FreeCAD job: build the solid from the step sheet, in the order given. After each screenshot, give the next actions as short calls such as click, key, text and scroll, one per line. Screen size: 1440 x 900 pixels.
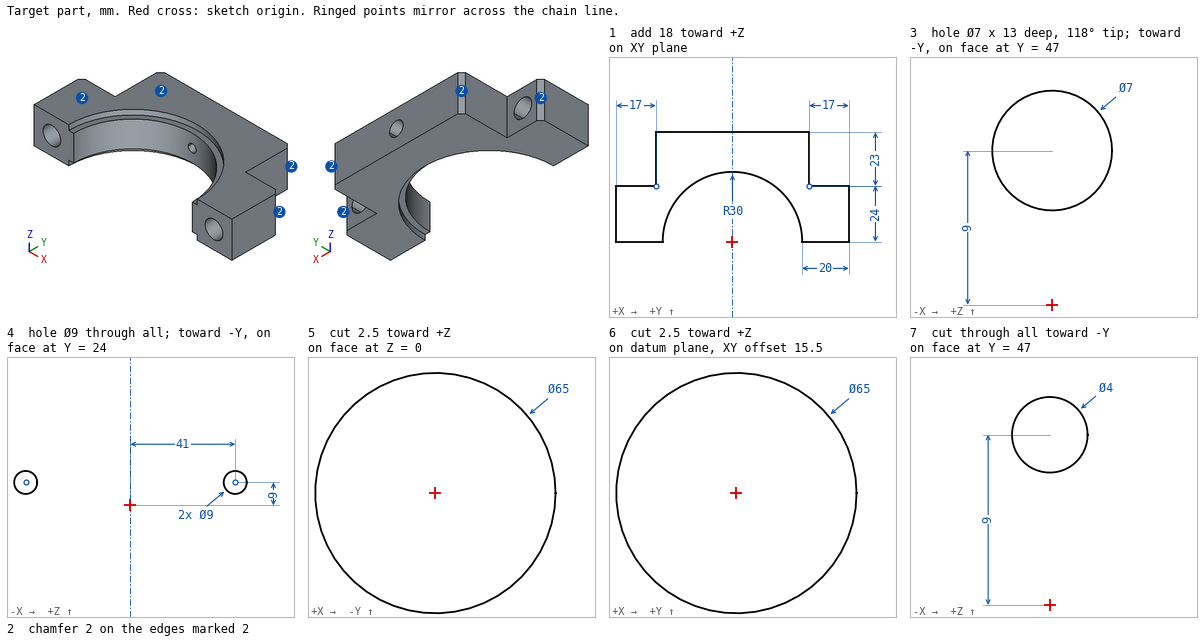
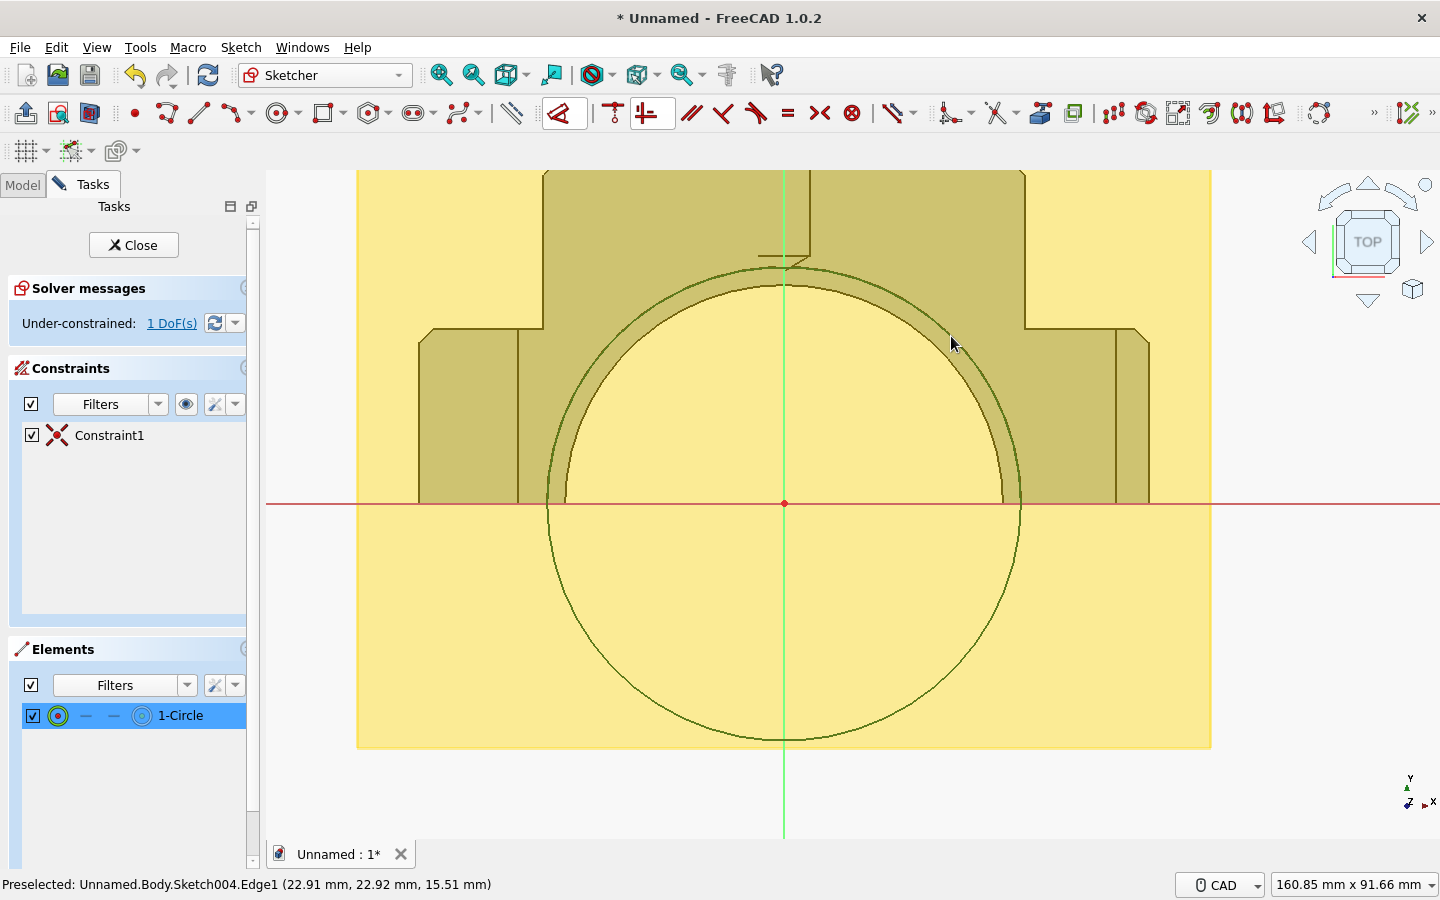
click(582, 114)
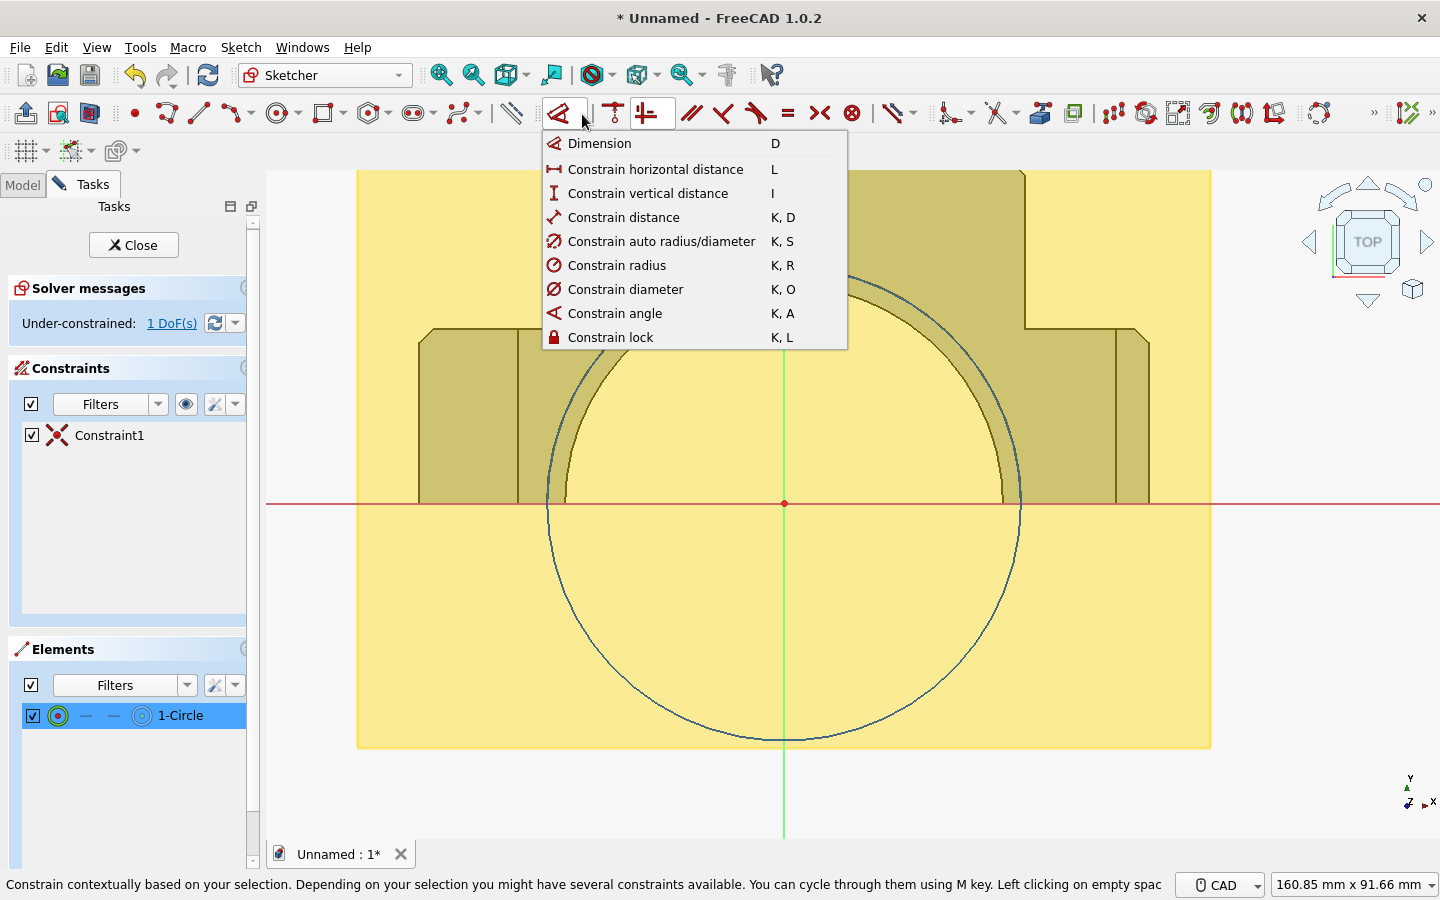
click(695, 289)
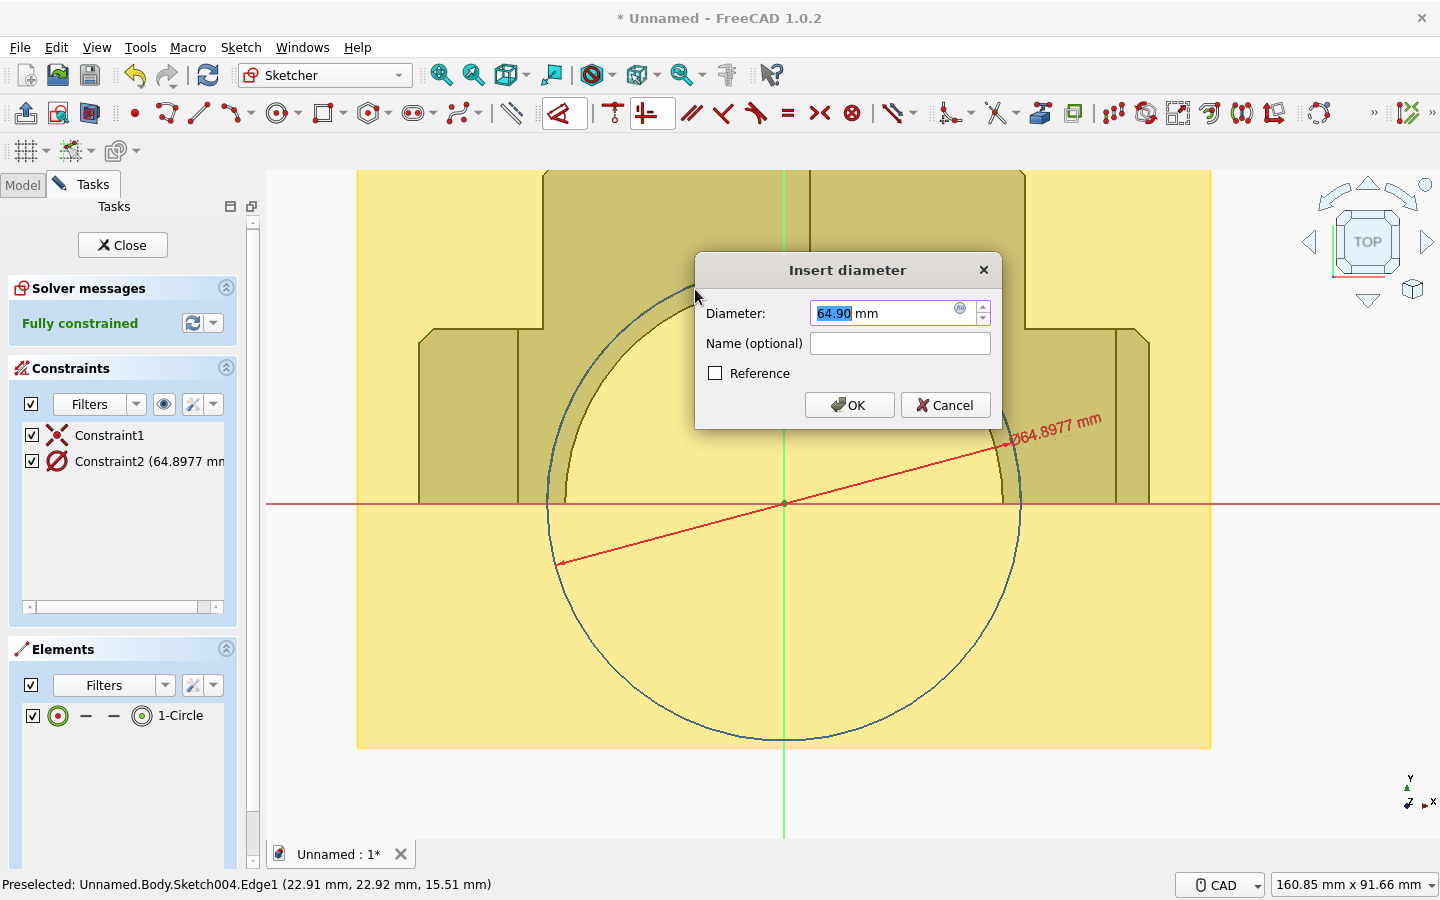
text(65)
key(Return)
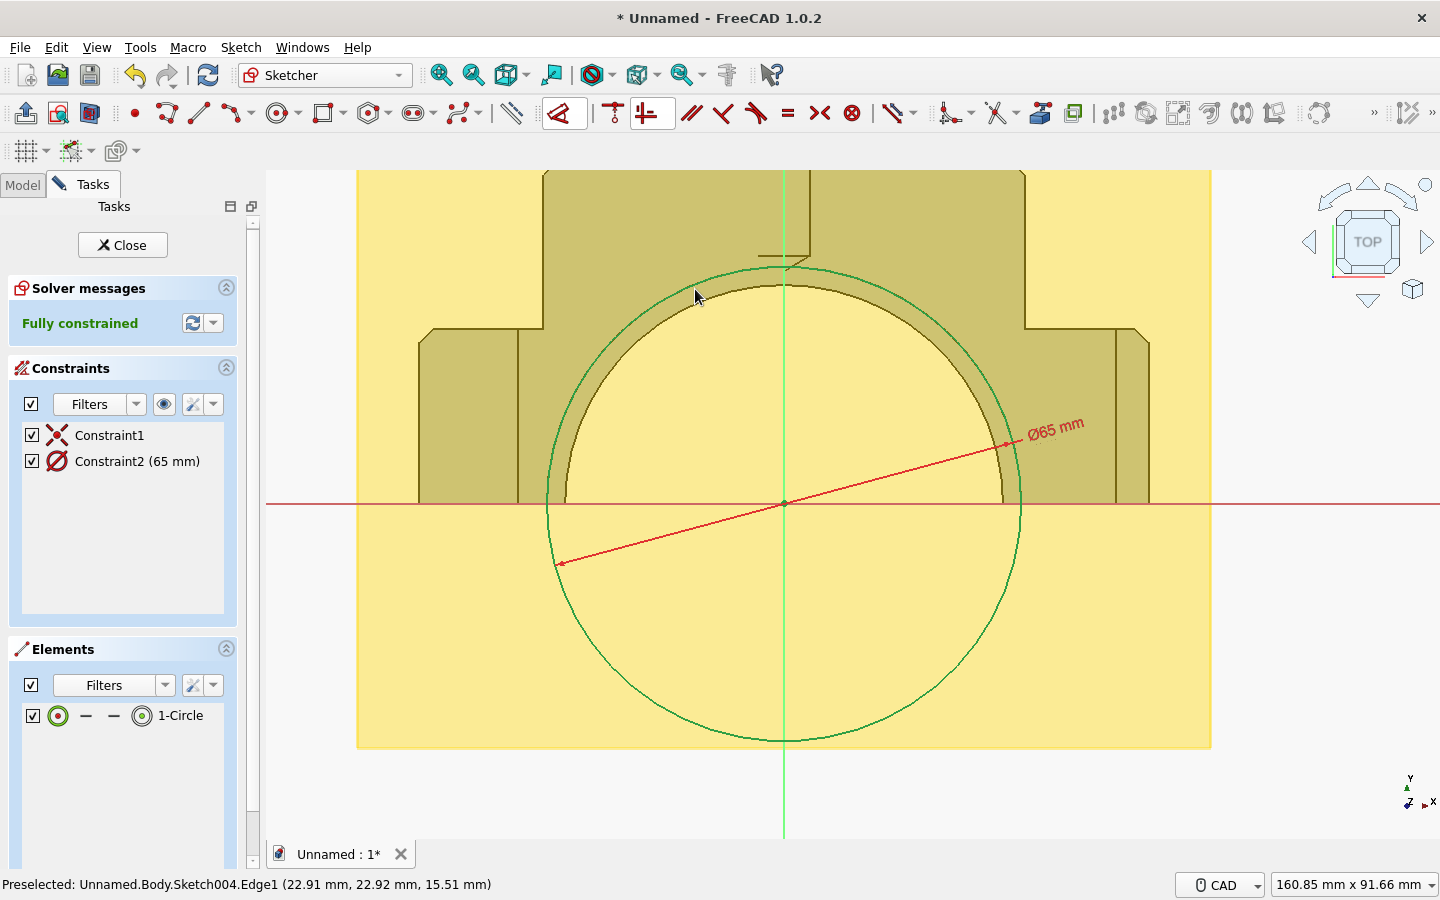
click(123, 245)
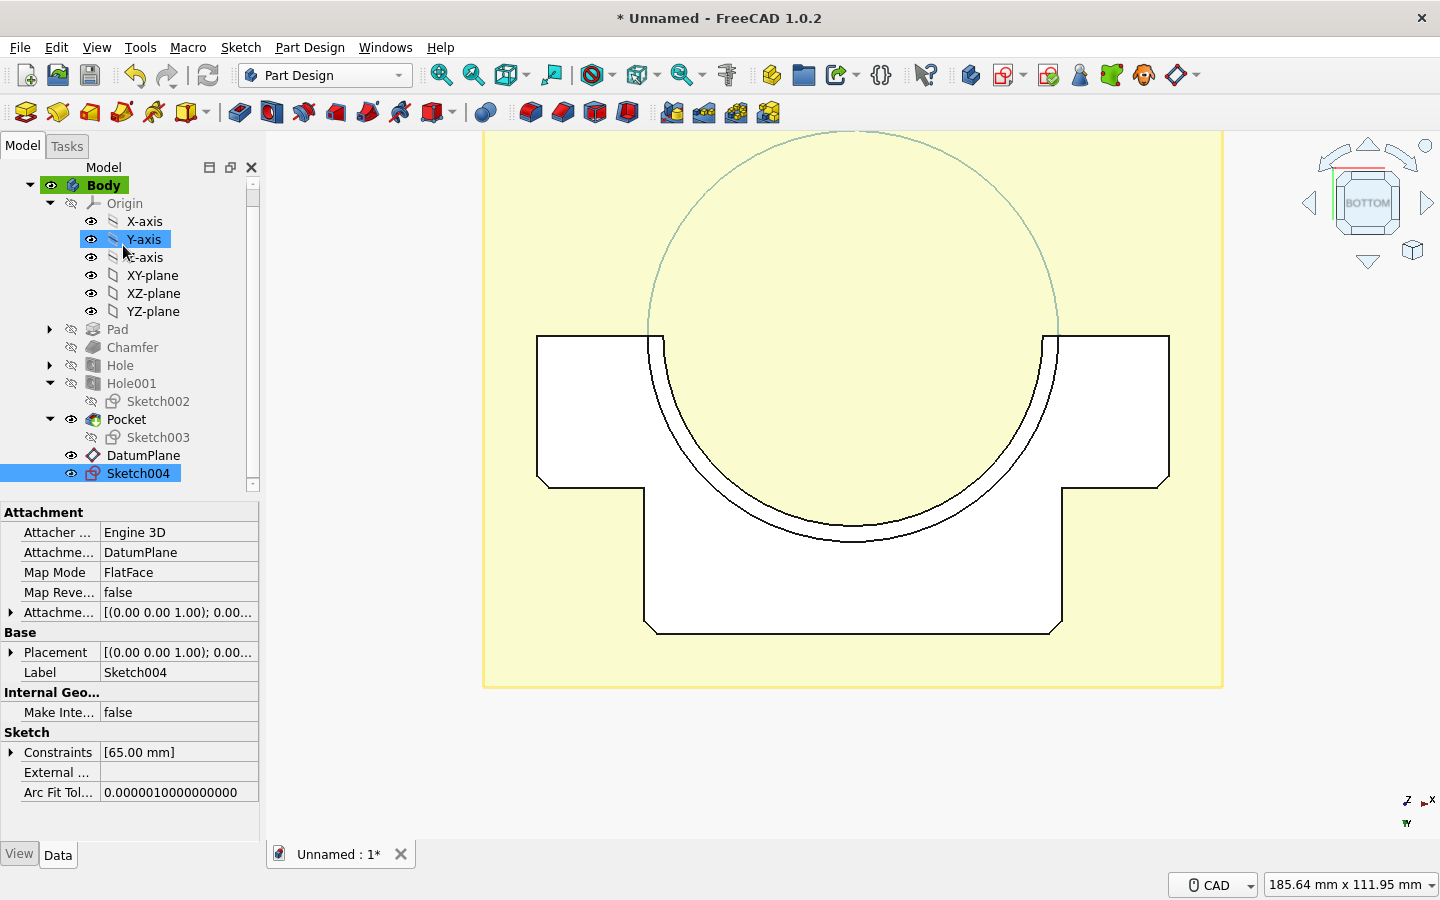
click(240, 112)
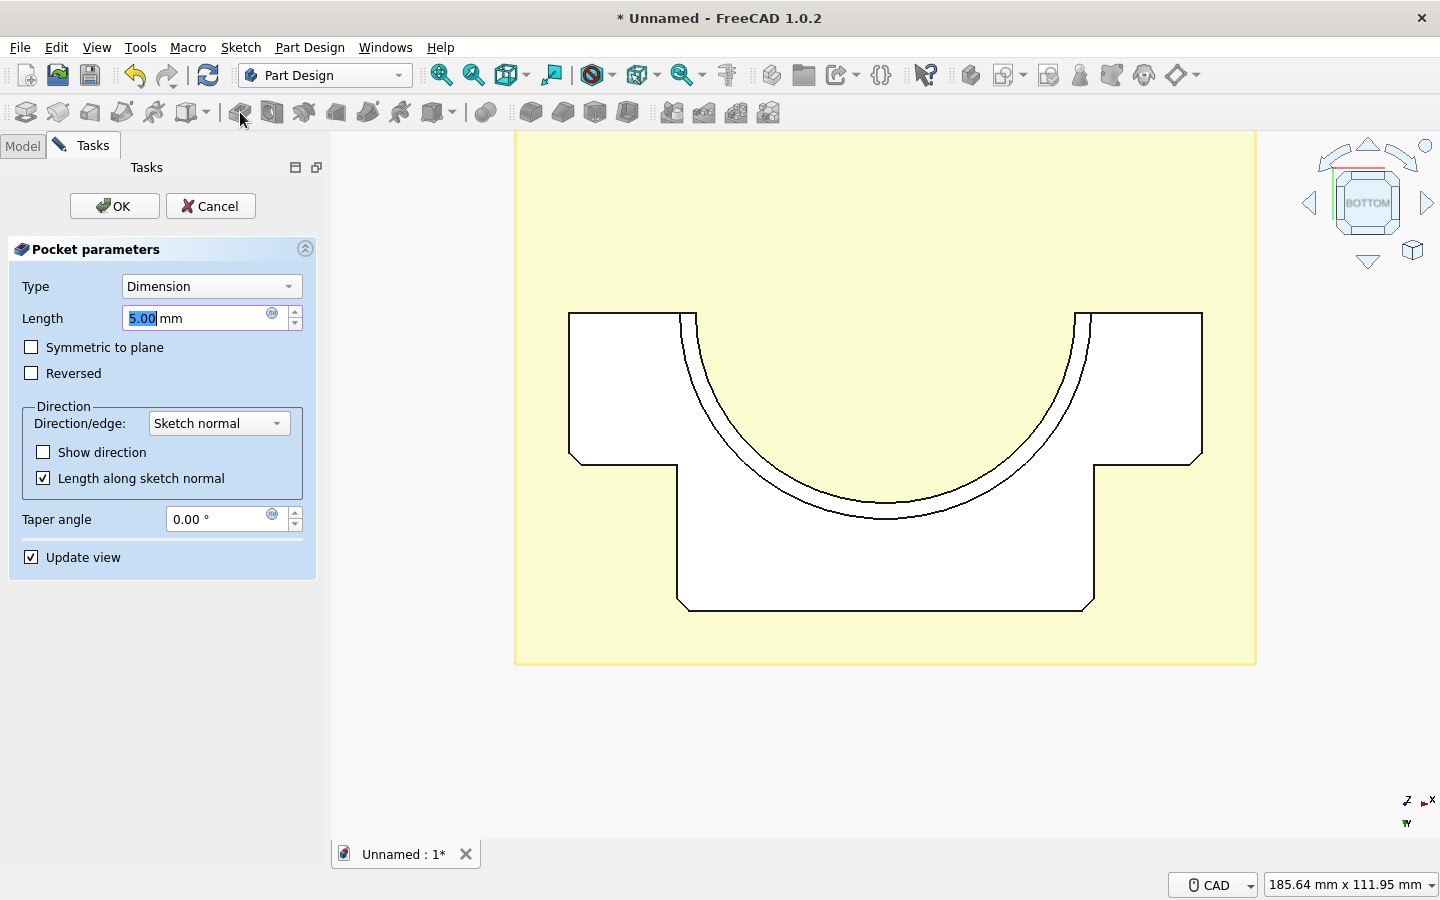
text(2.5)
key(Tab)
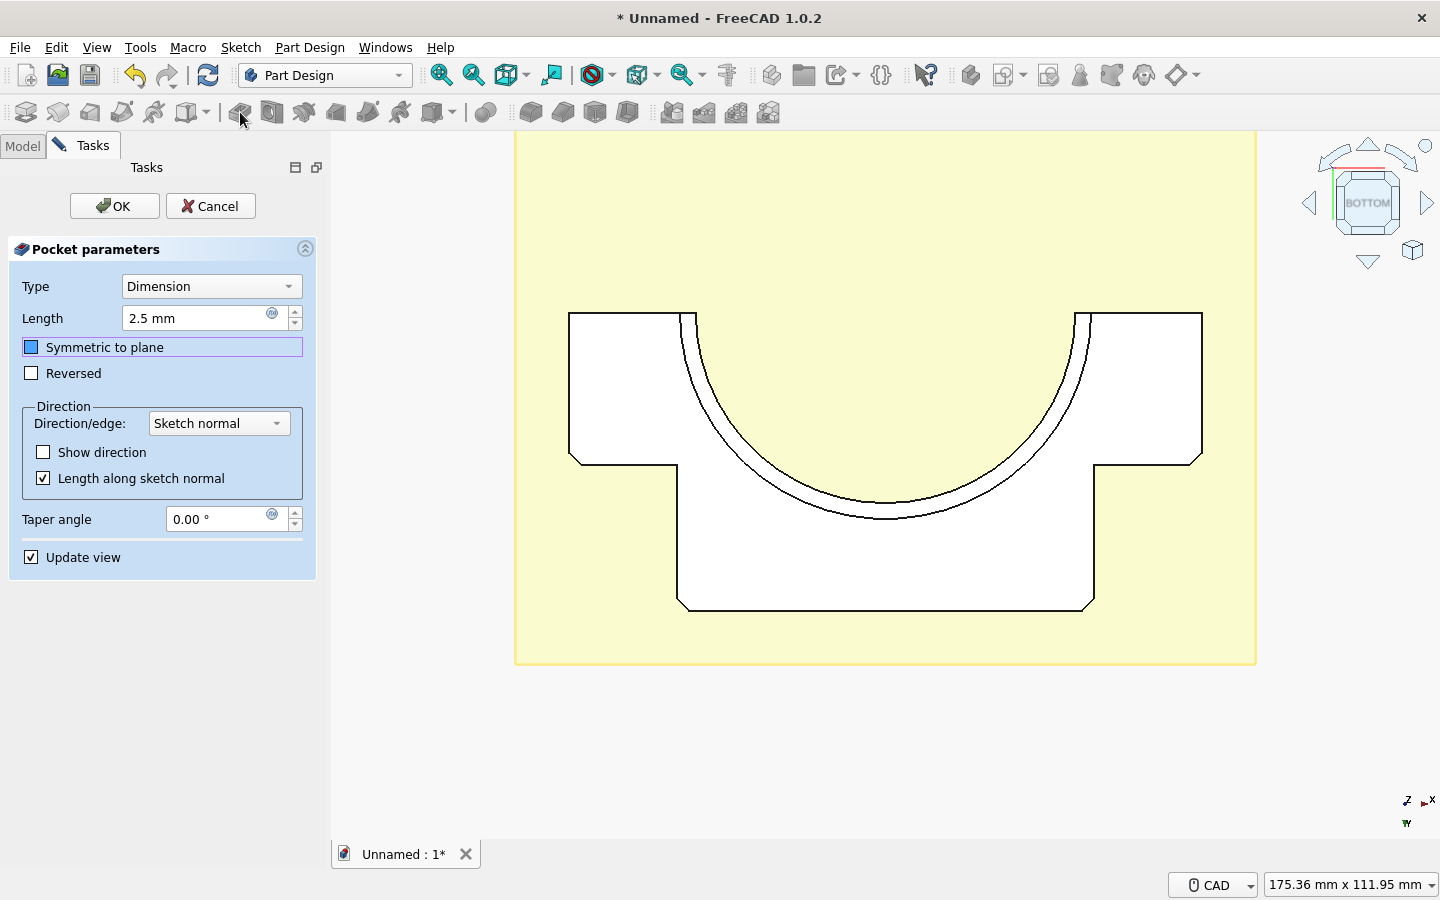
click(30, 373)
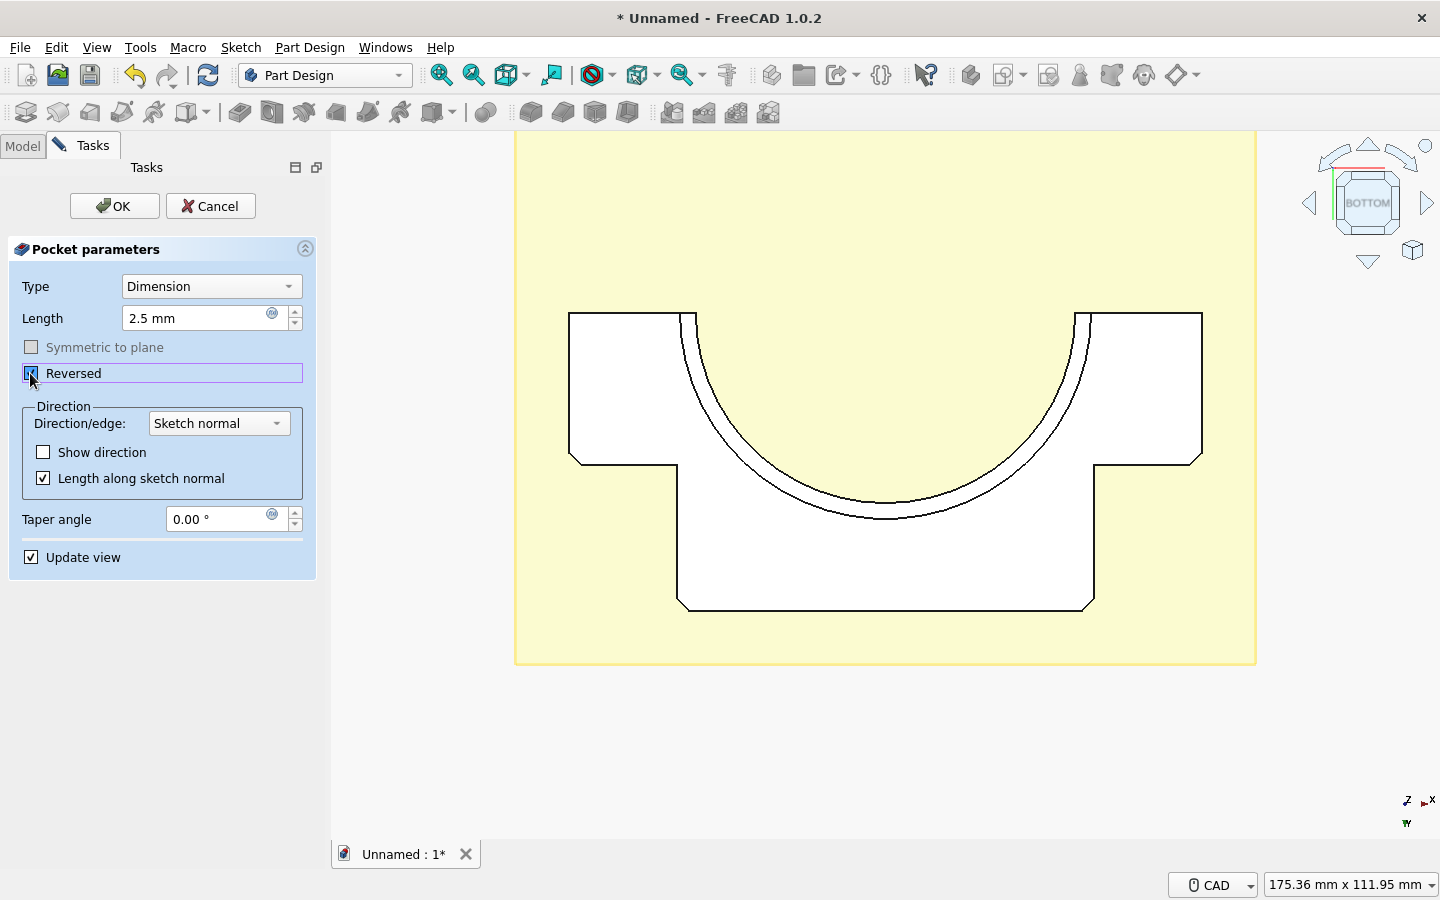
click(115, 206)